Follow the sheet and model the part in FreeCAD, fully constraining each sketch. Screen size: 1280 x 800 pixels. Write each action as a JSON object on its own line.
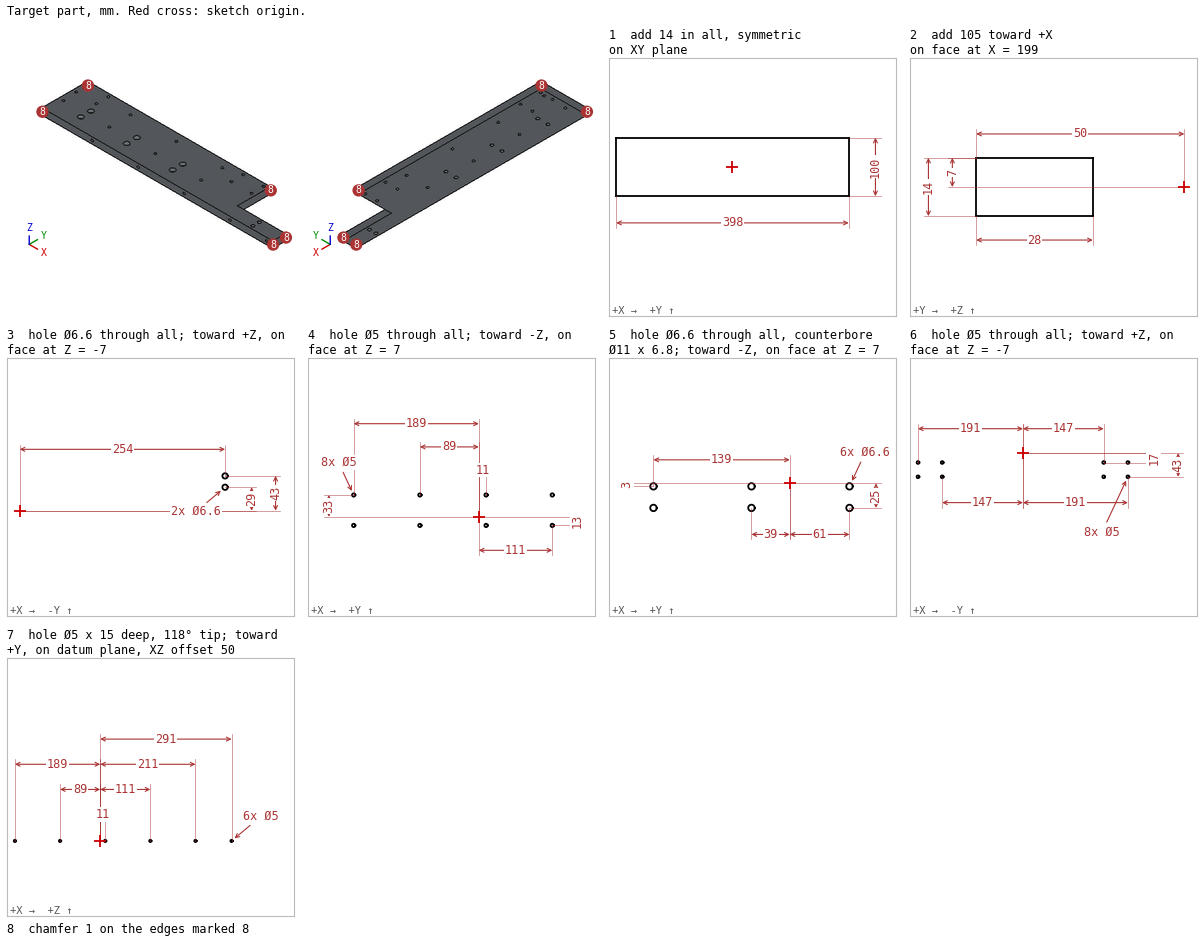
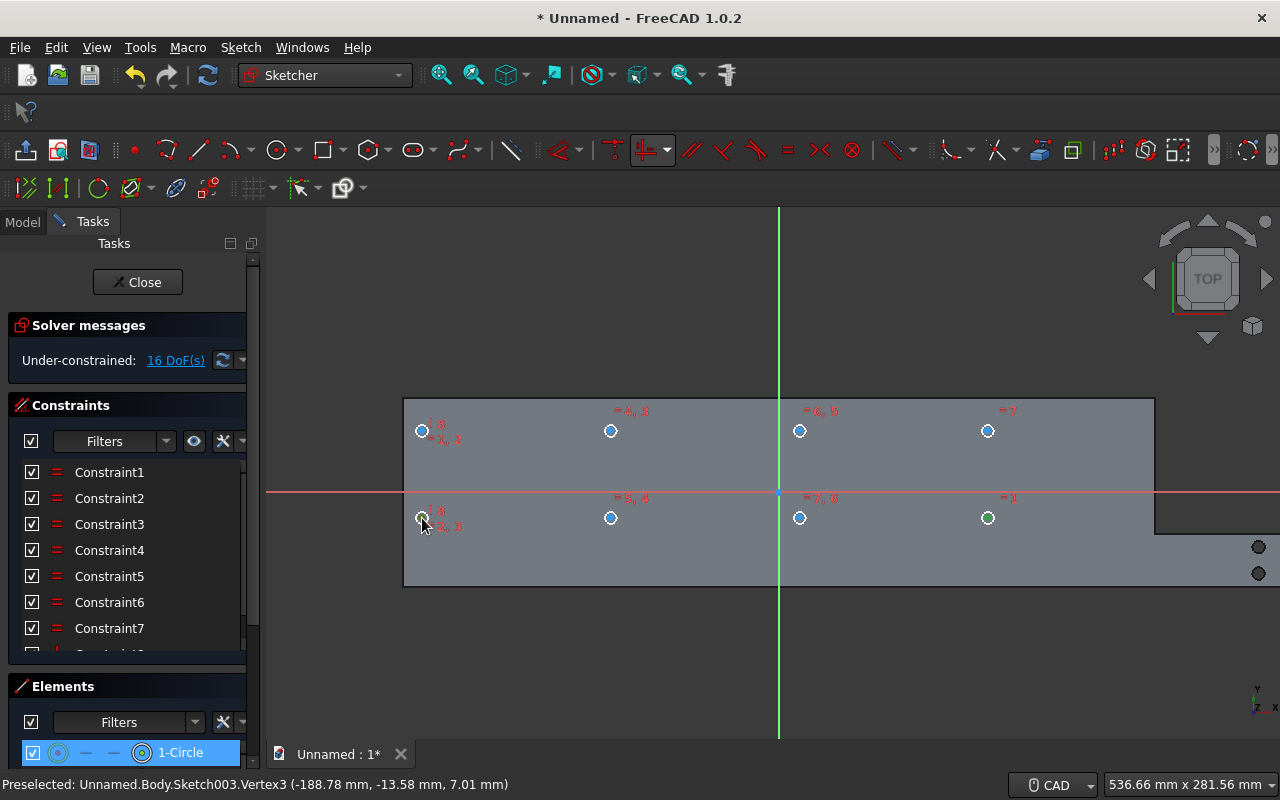
{"action": "key", "text": "h"}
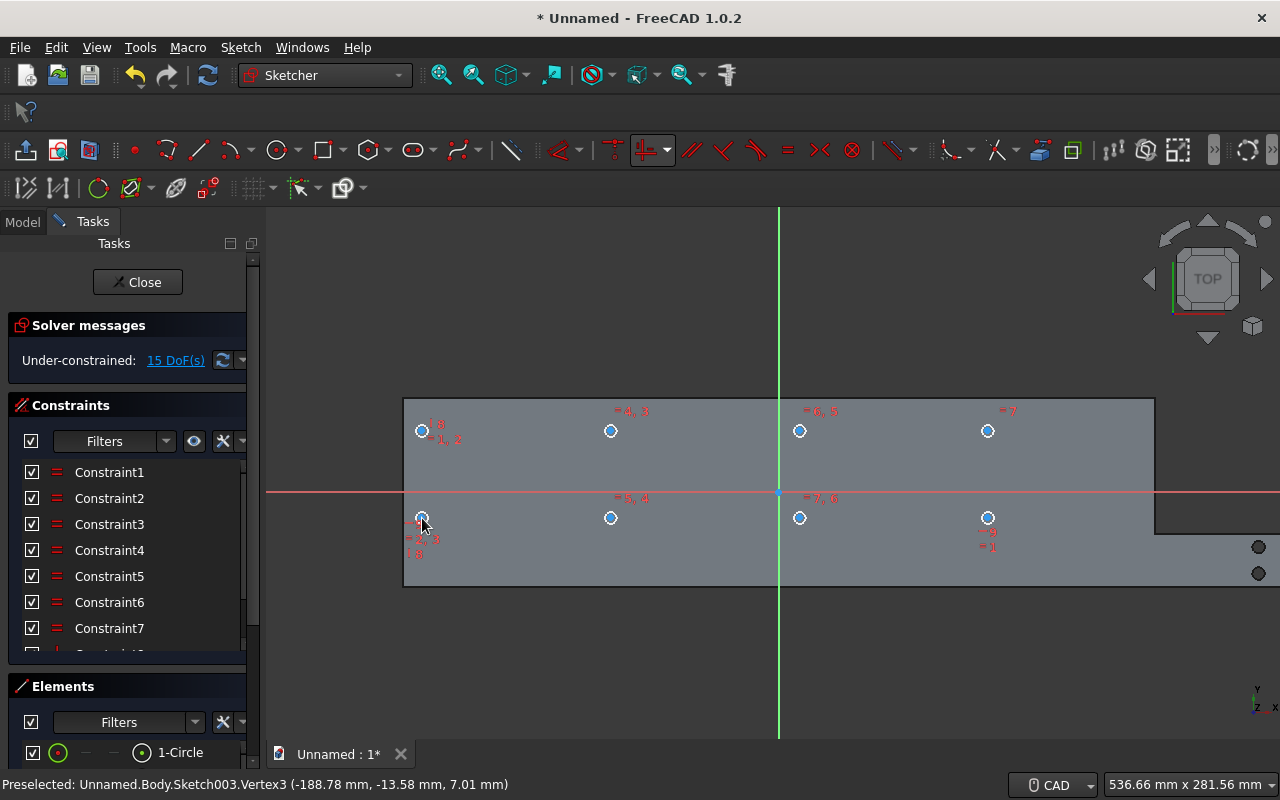
{"action": "left_click", "coordinate": [422, 431]}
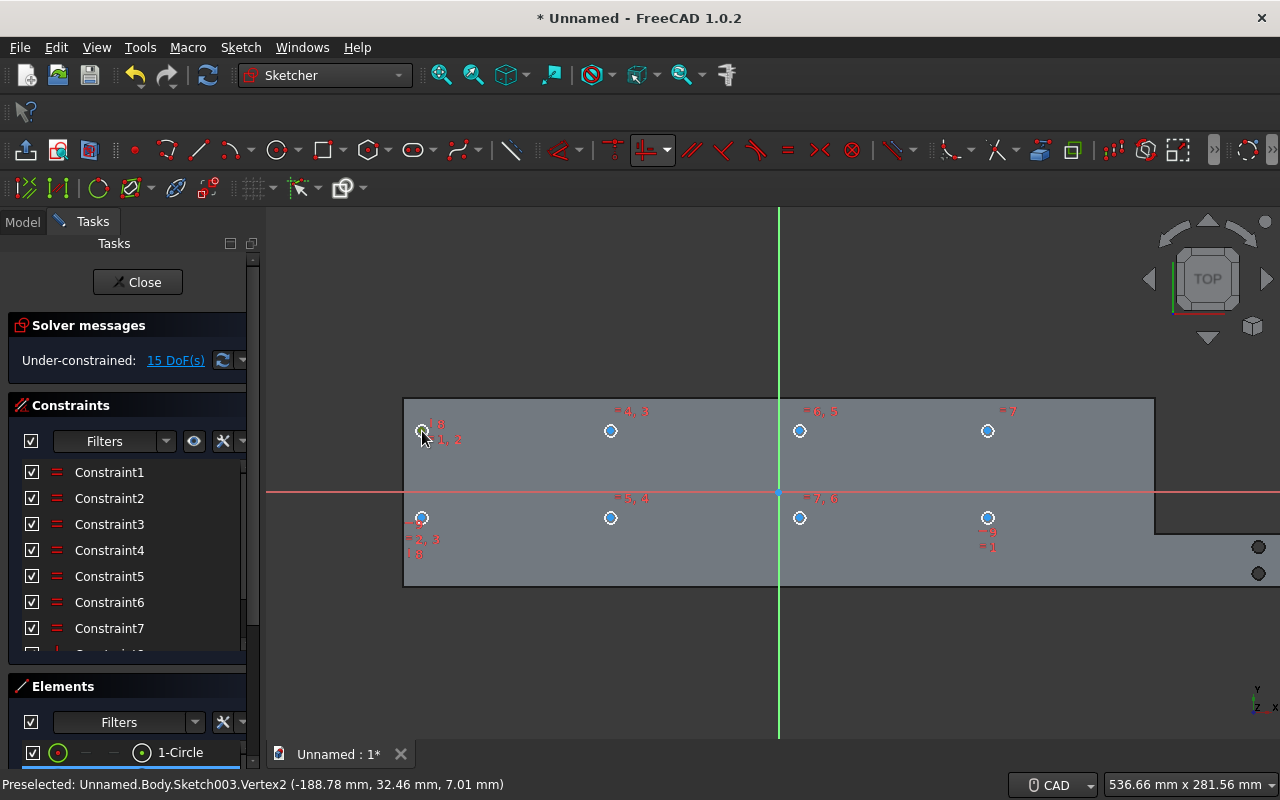
{"action": "left_click", "coordinate": [611, 431]}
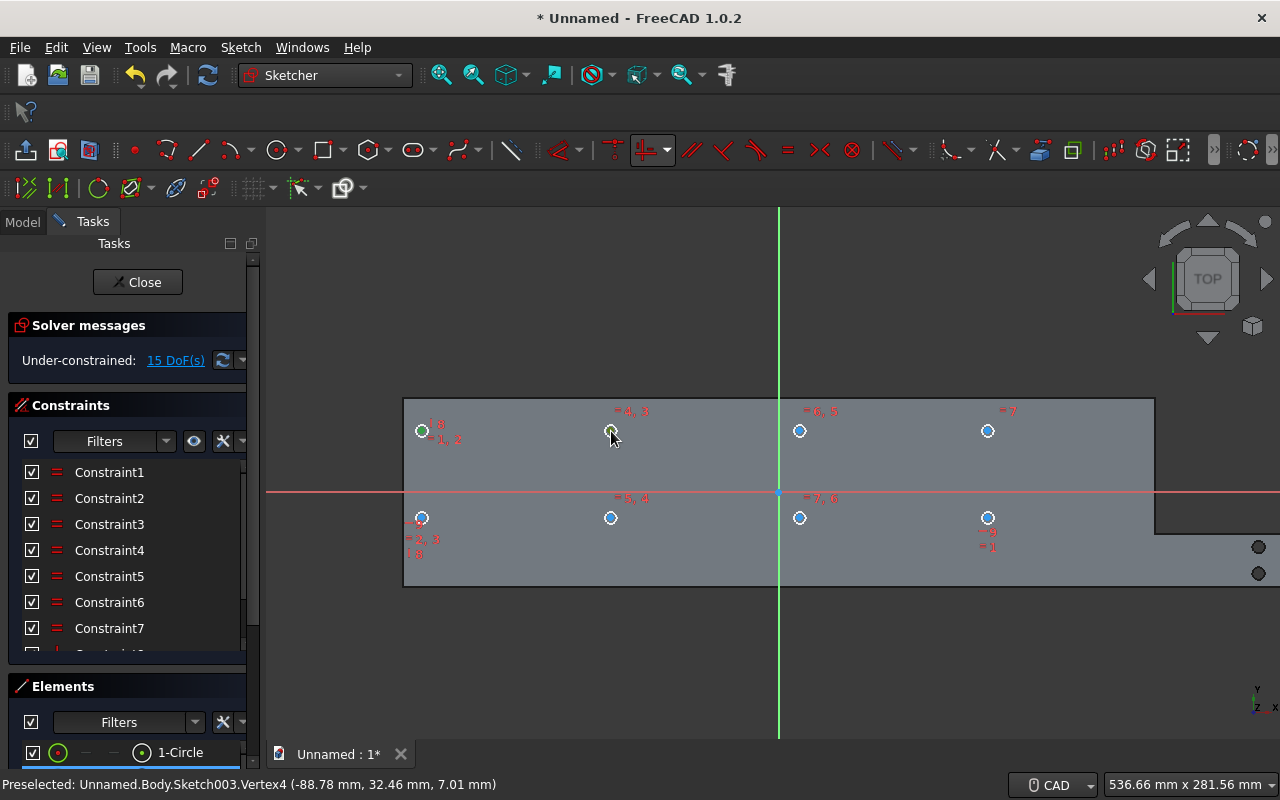
{"action": "key", "text": "h"}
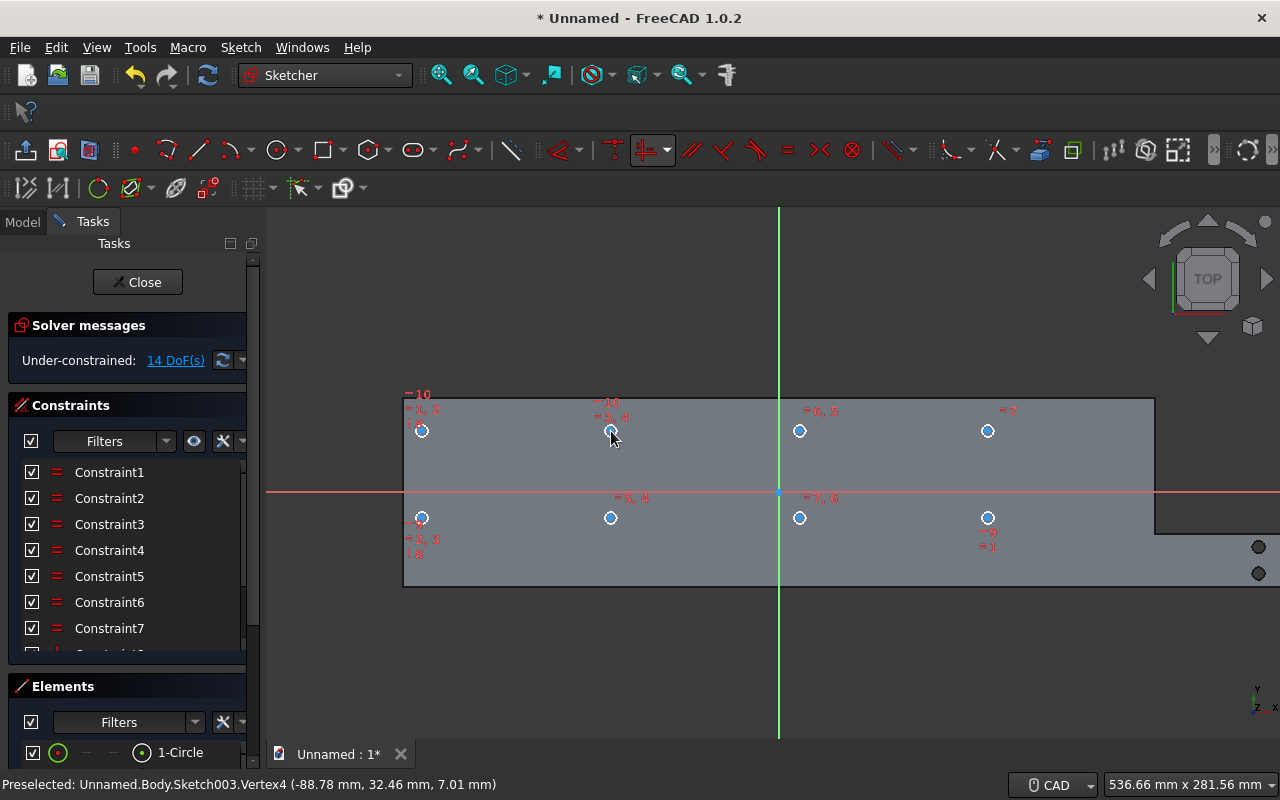
{"action": "left_click", "coordinate": [611, 431]}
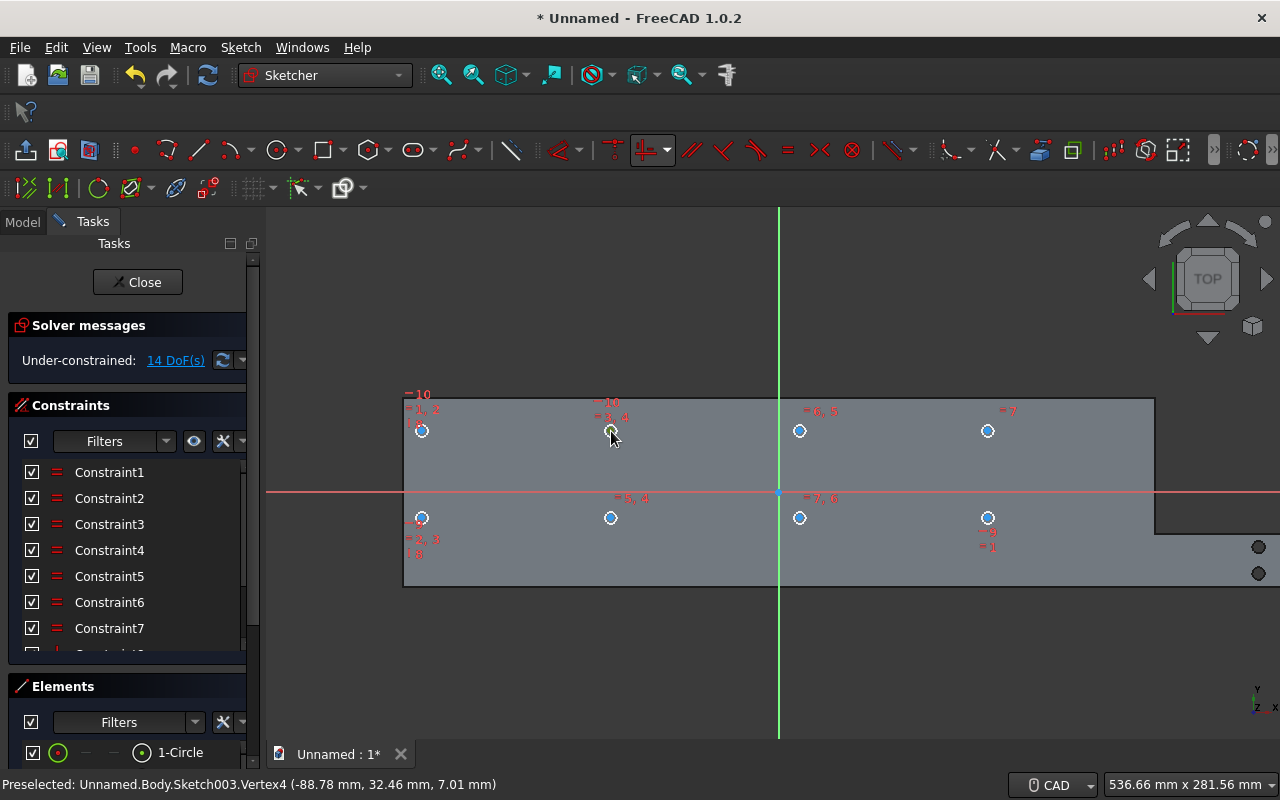
{"action": "left_click", "coordinate": [611, 518]}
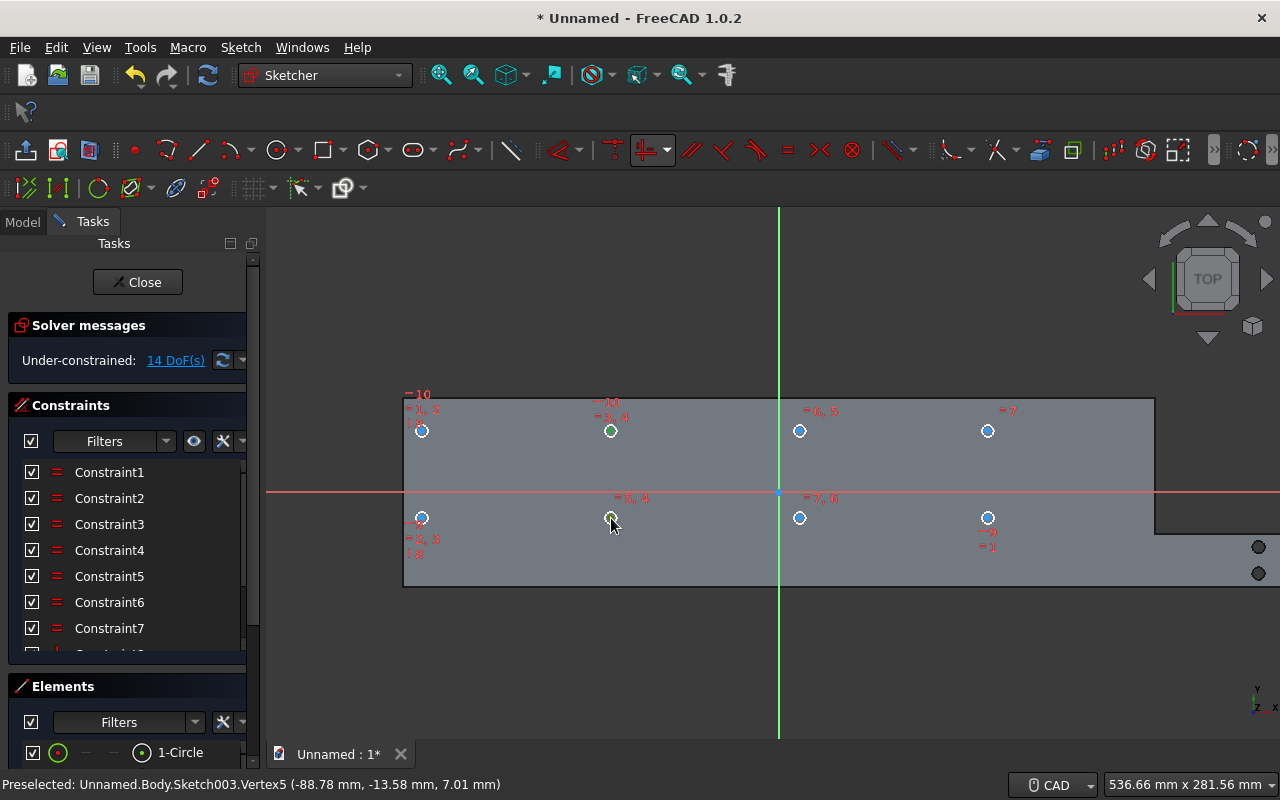
{"action": "key", "text": "v"}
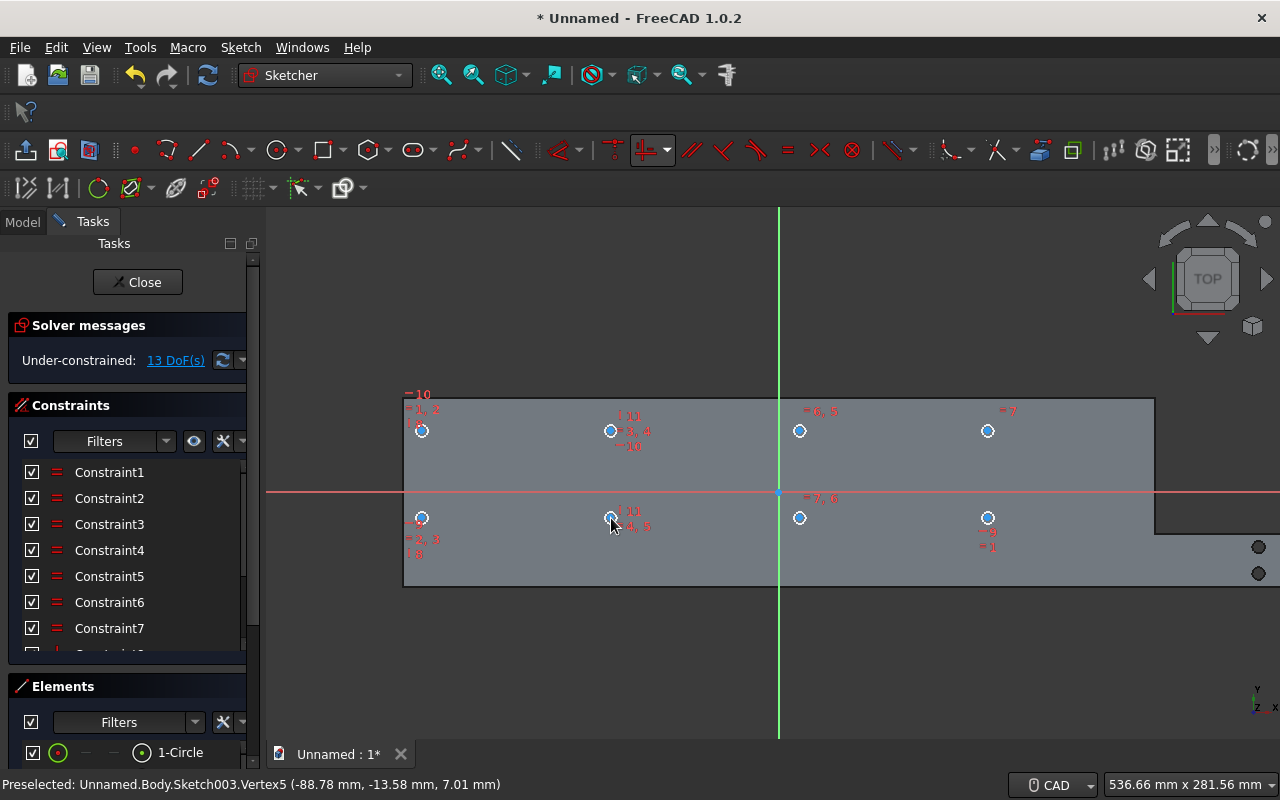
{"action": "scroll", "coordinate": [422, 518], "scroll_direction": "up", "scroll_amount": 4}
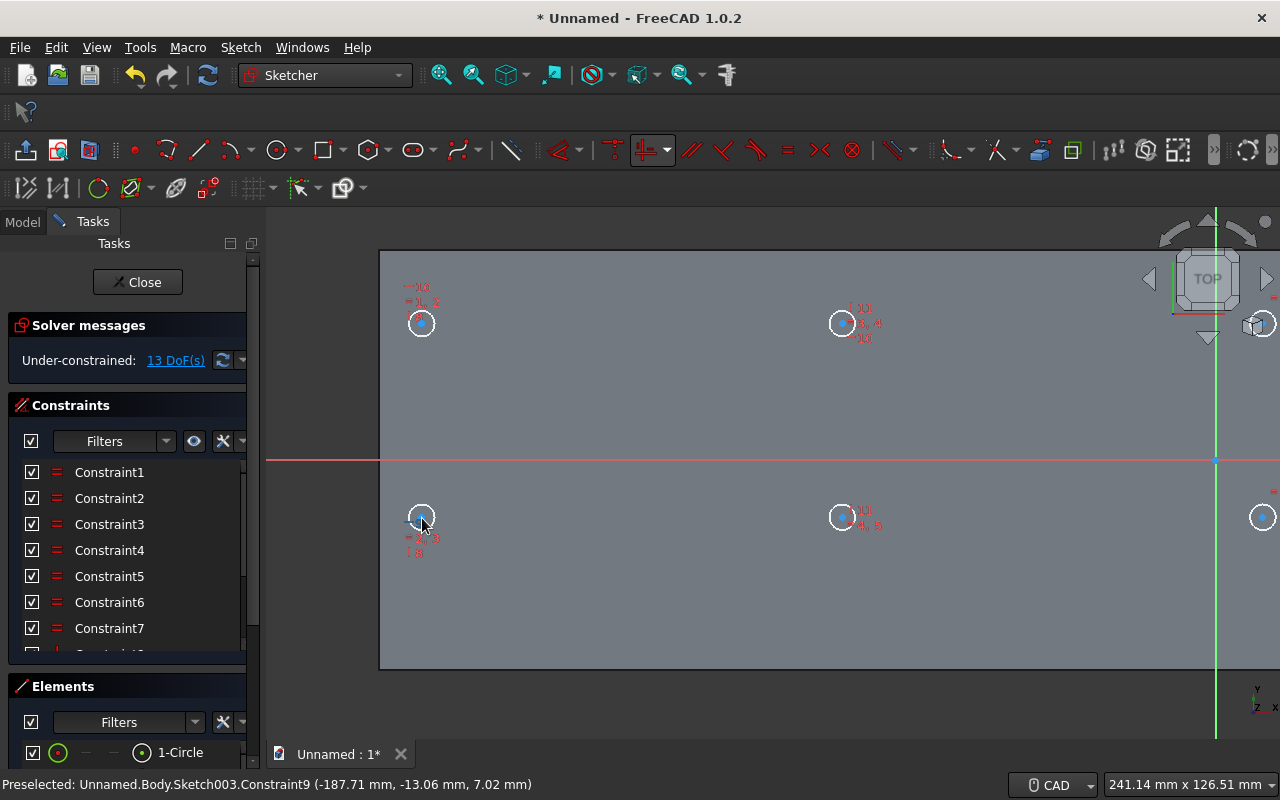
{"action": "left_click", "coordinate": [420, 515]}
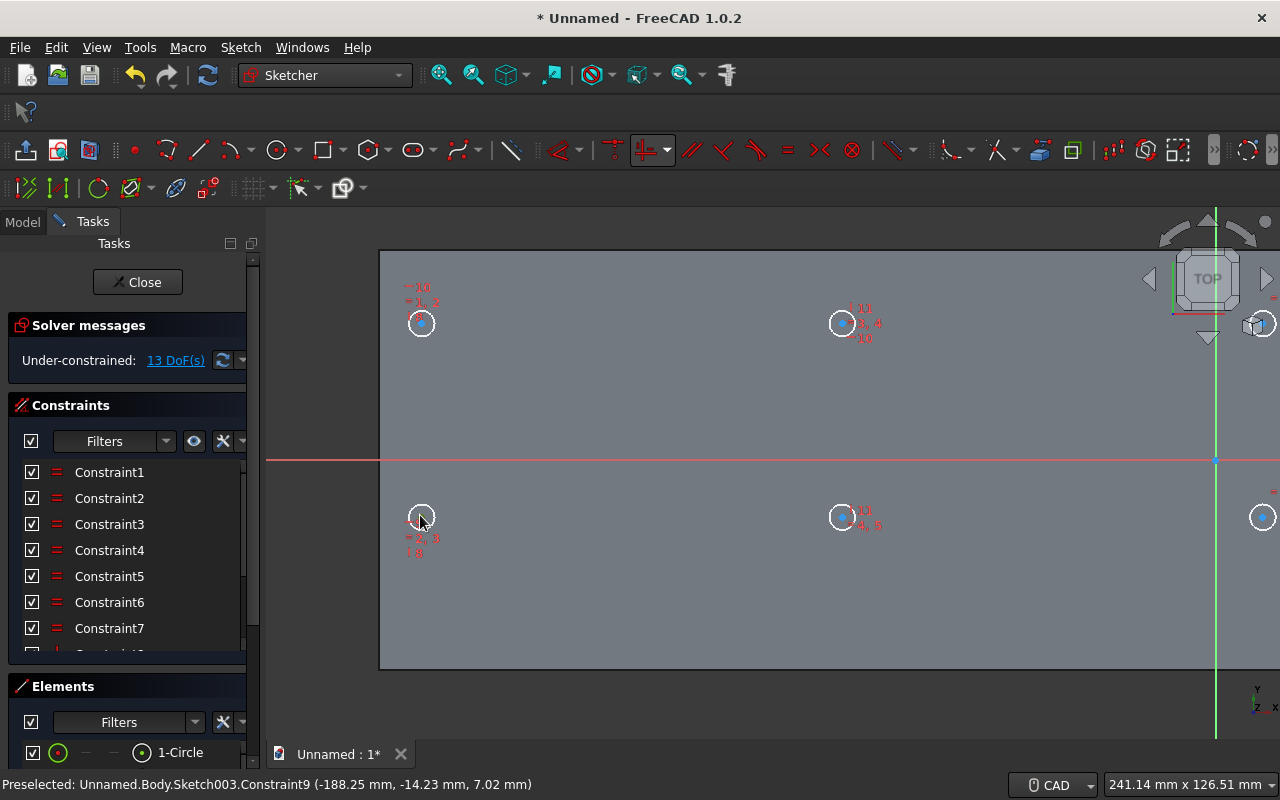
{"action": "left_click", "coordinate": [842, 517]}